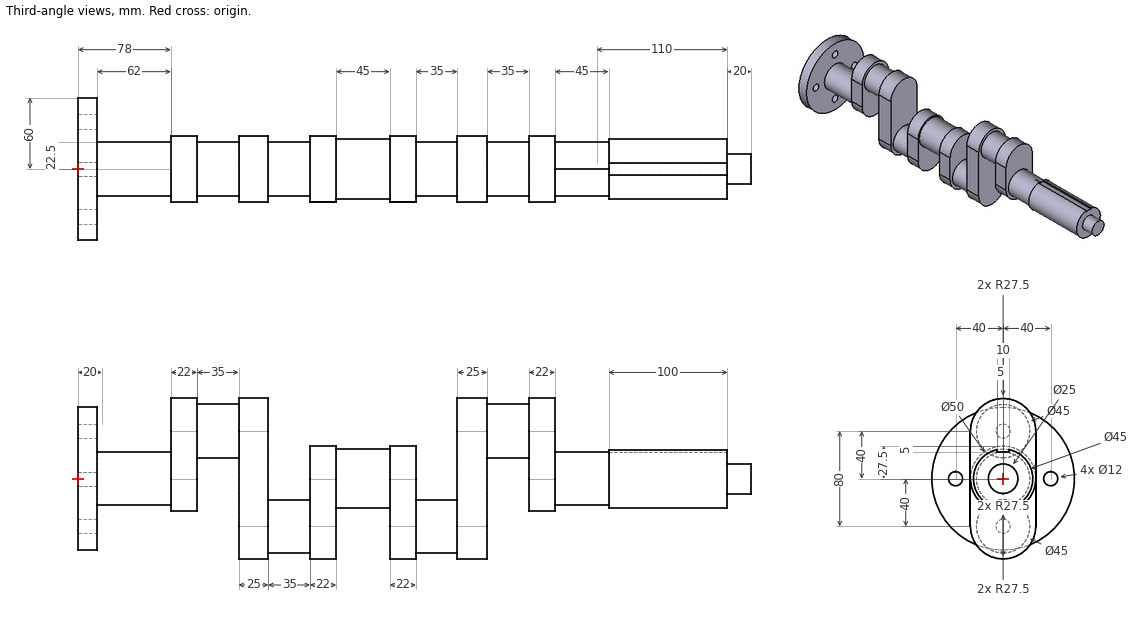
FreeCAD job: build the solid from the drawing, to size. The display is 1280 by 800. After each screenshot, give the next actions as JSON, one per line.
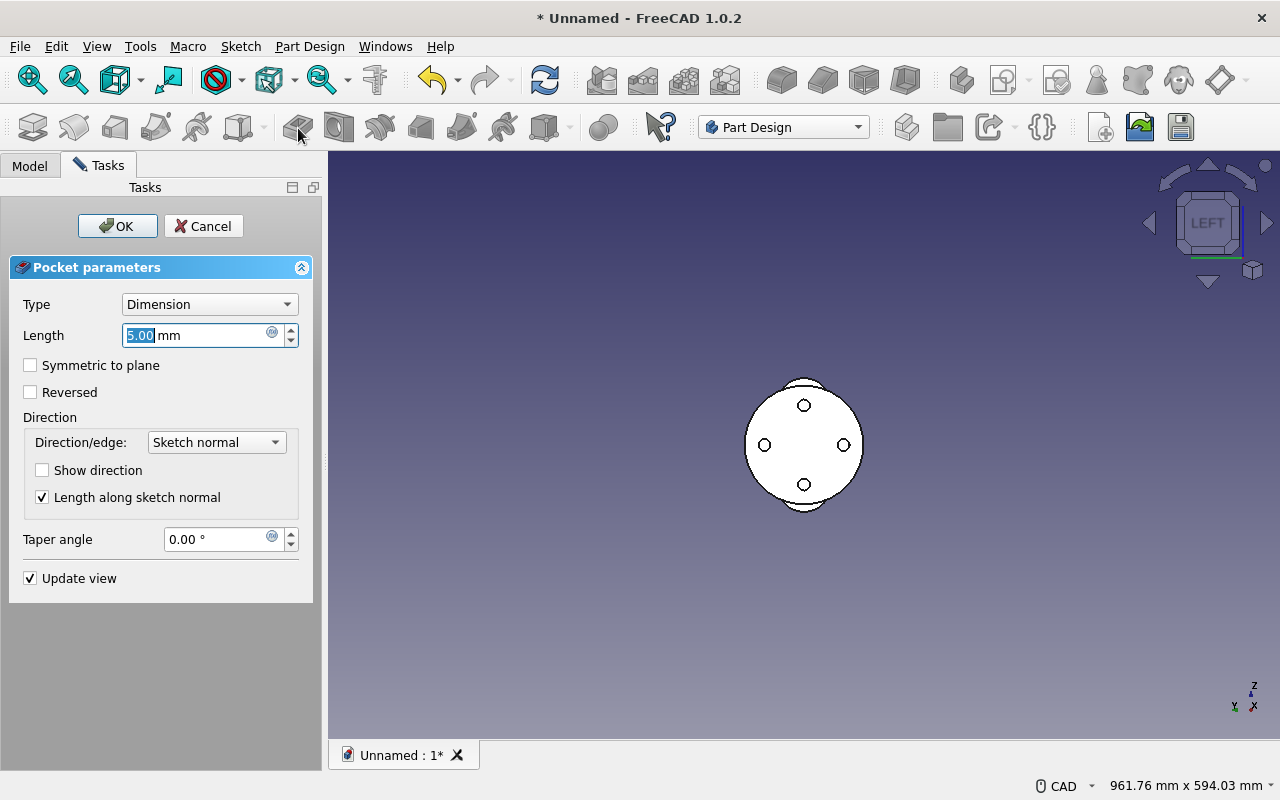
{"action": "type", "text": "20"}
{"action": "key", "text": "Tab"}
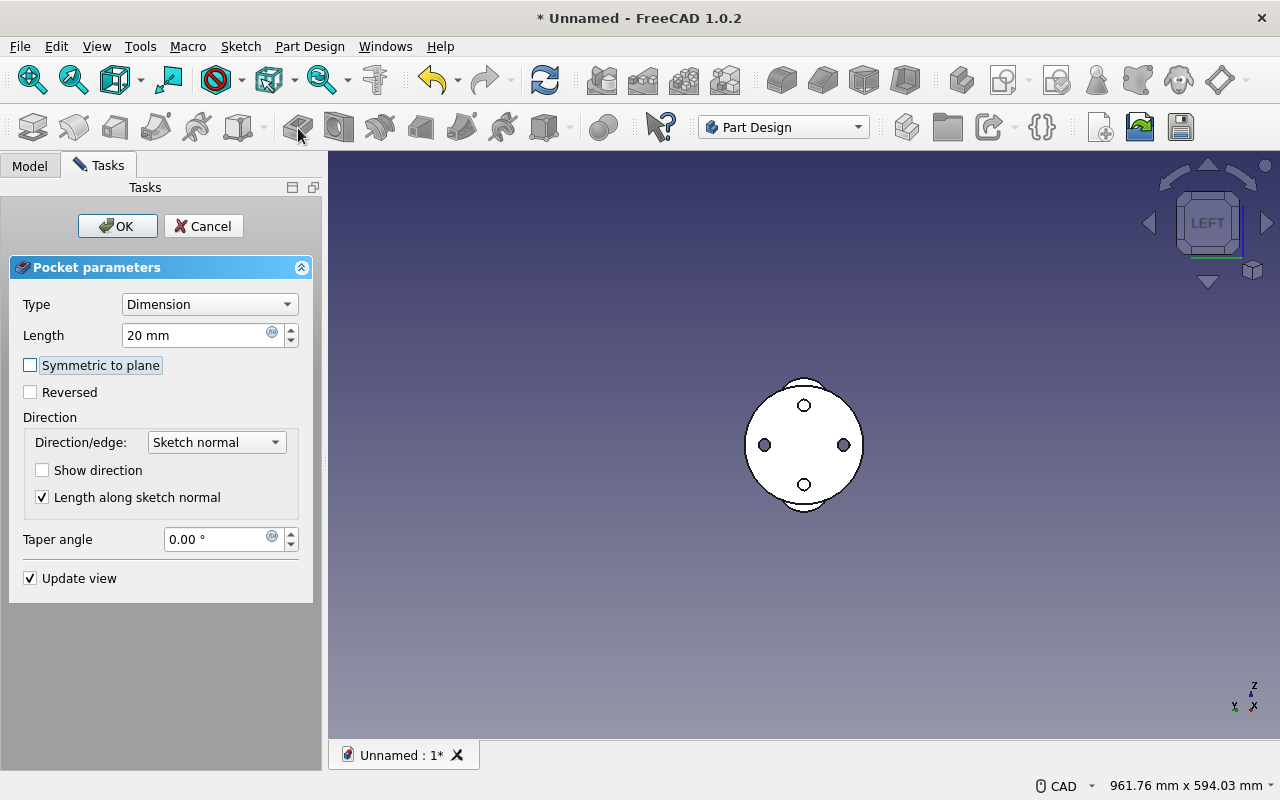
{"action": "left_click", "coordinate": [118, 226]}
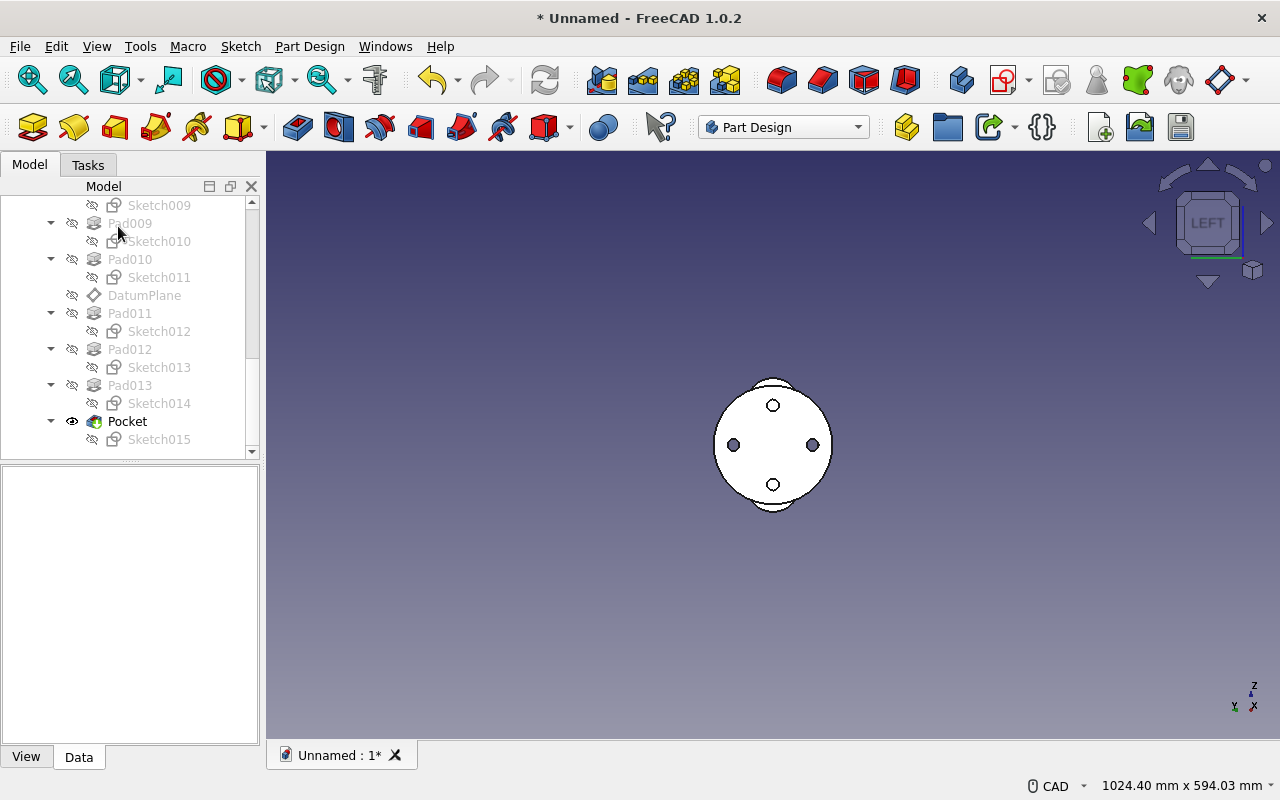
{"action": "left_click", "coordinate": [33, 80]}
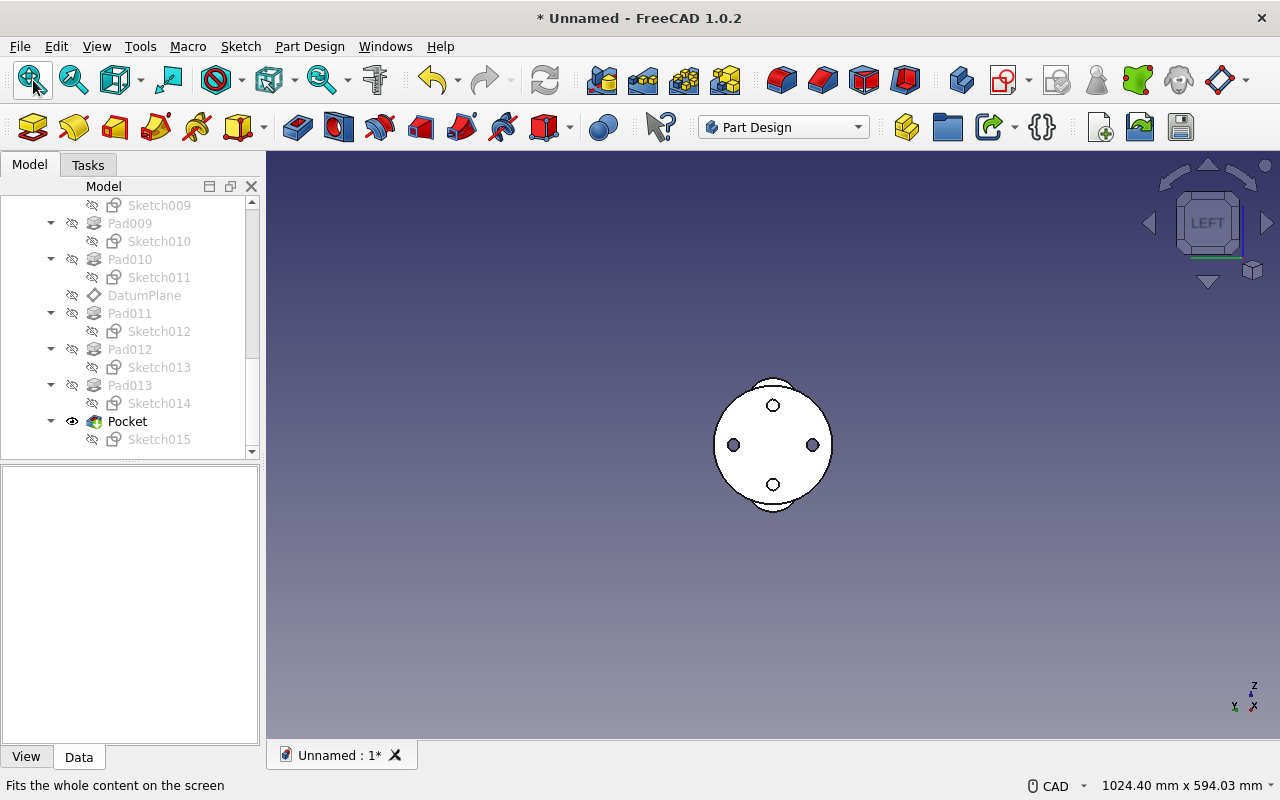
{"action": "key", "text": "0"}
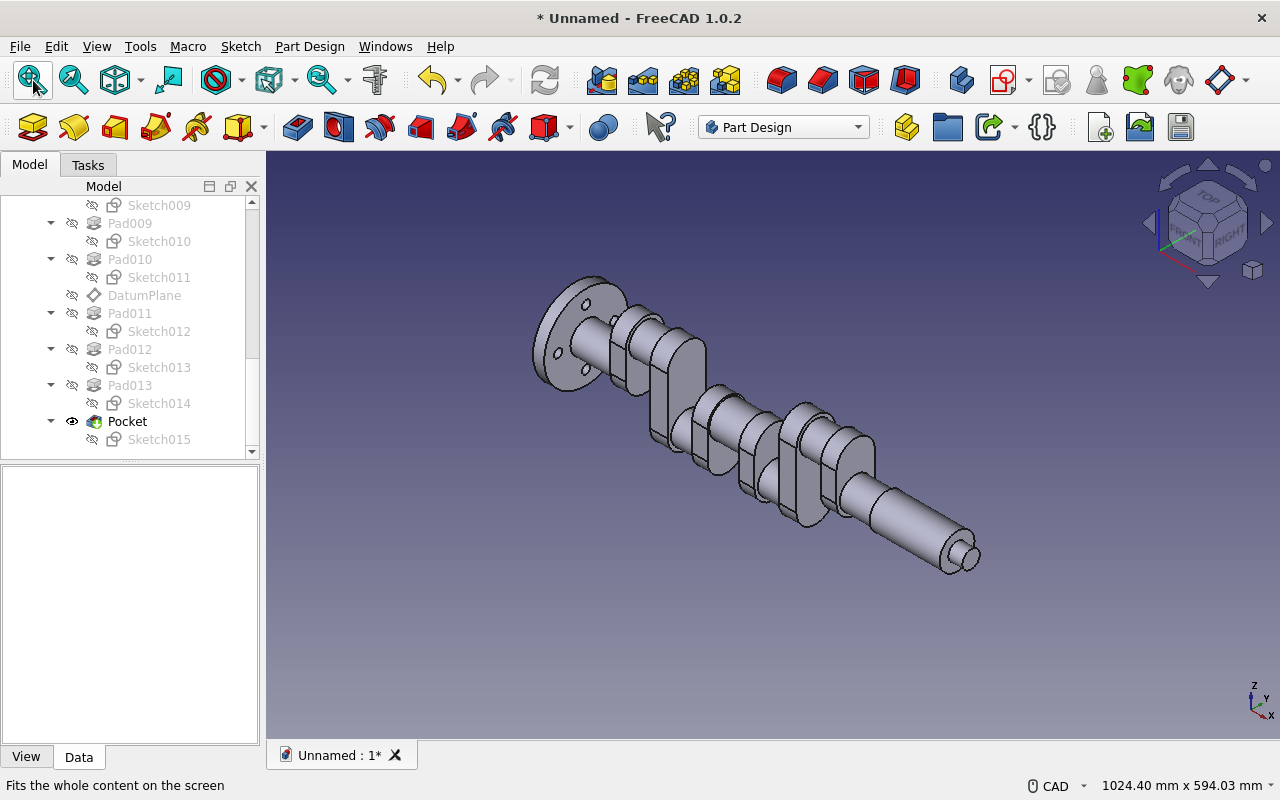
{"action": "scroll", "coordinate": [947, 568], "scroll_direction": "up", "scroll_amount": 5}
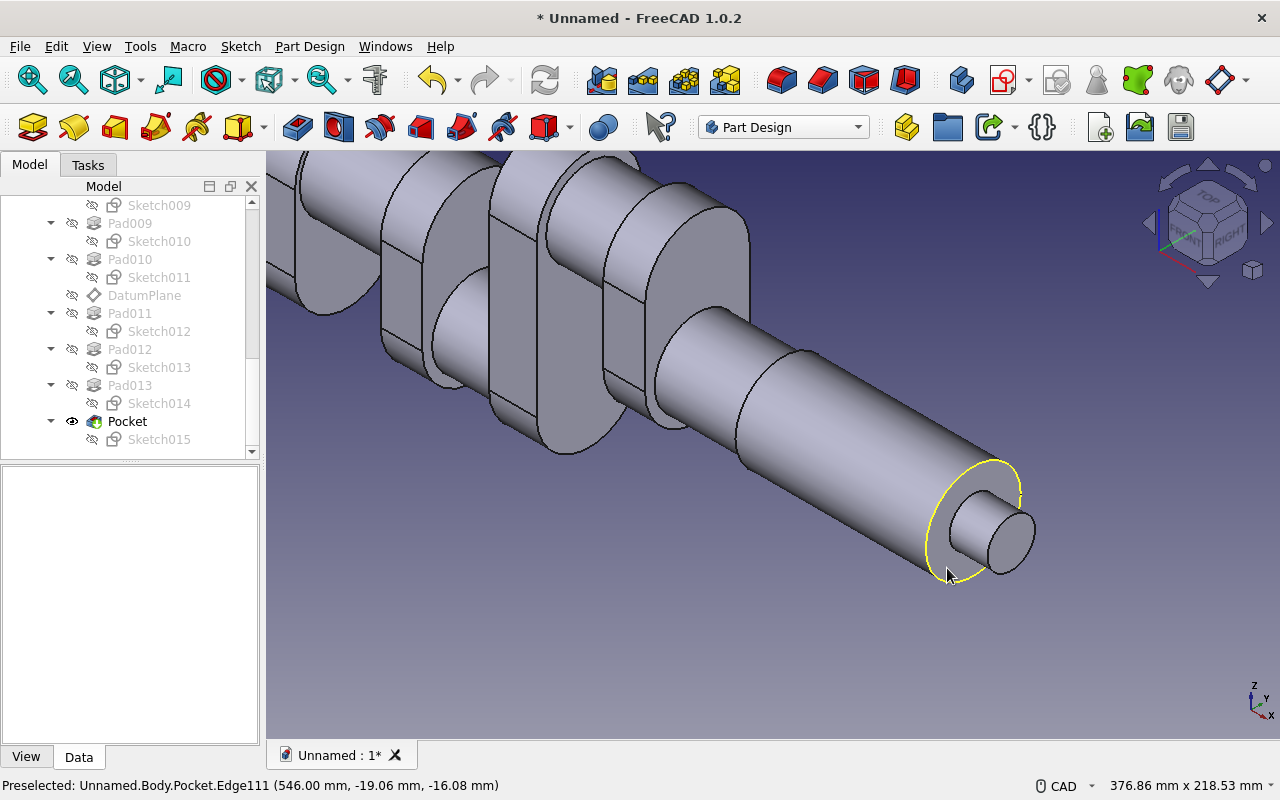
{"action": "left_click", "coordinate": [946, 567]}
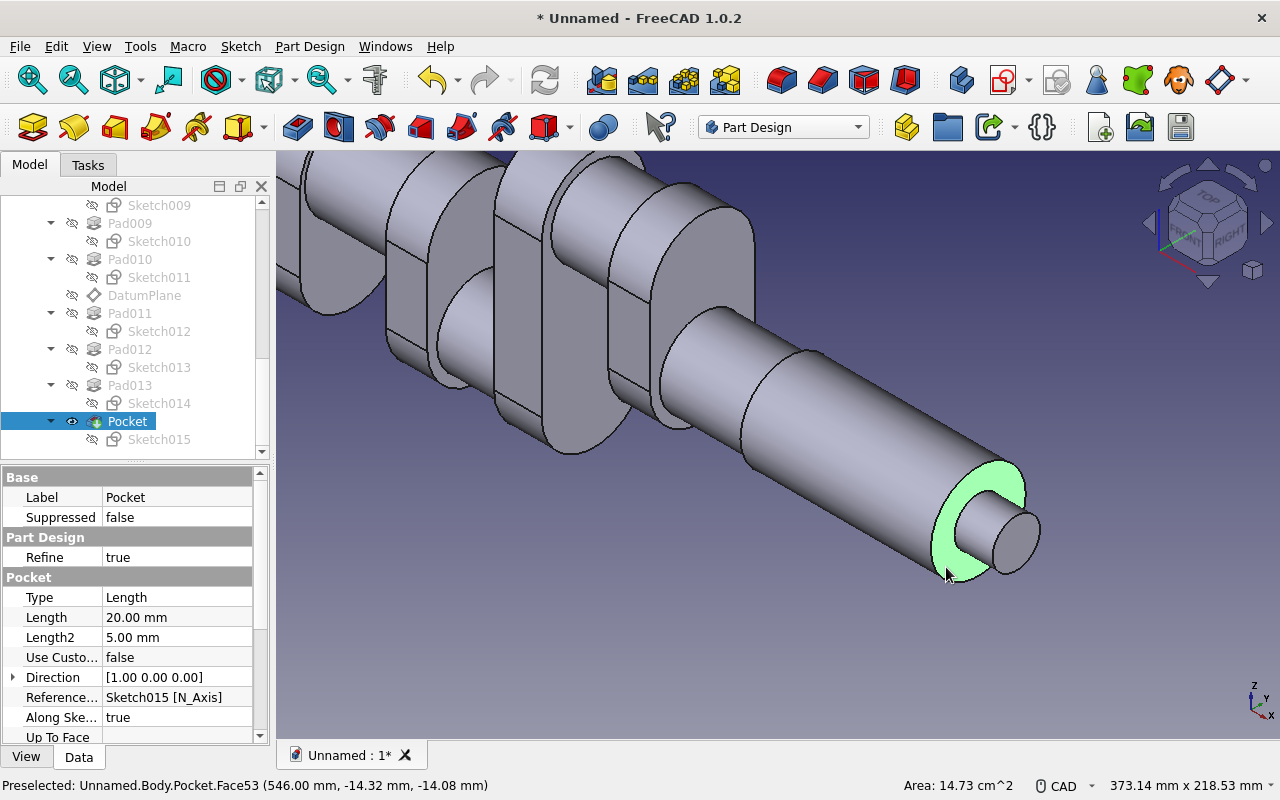
{"action": "left_click", "coordinate": [1002, 80]}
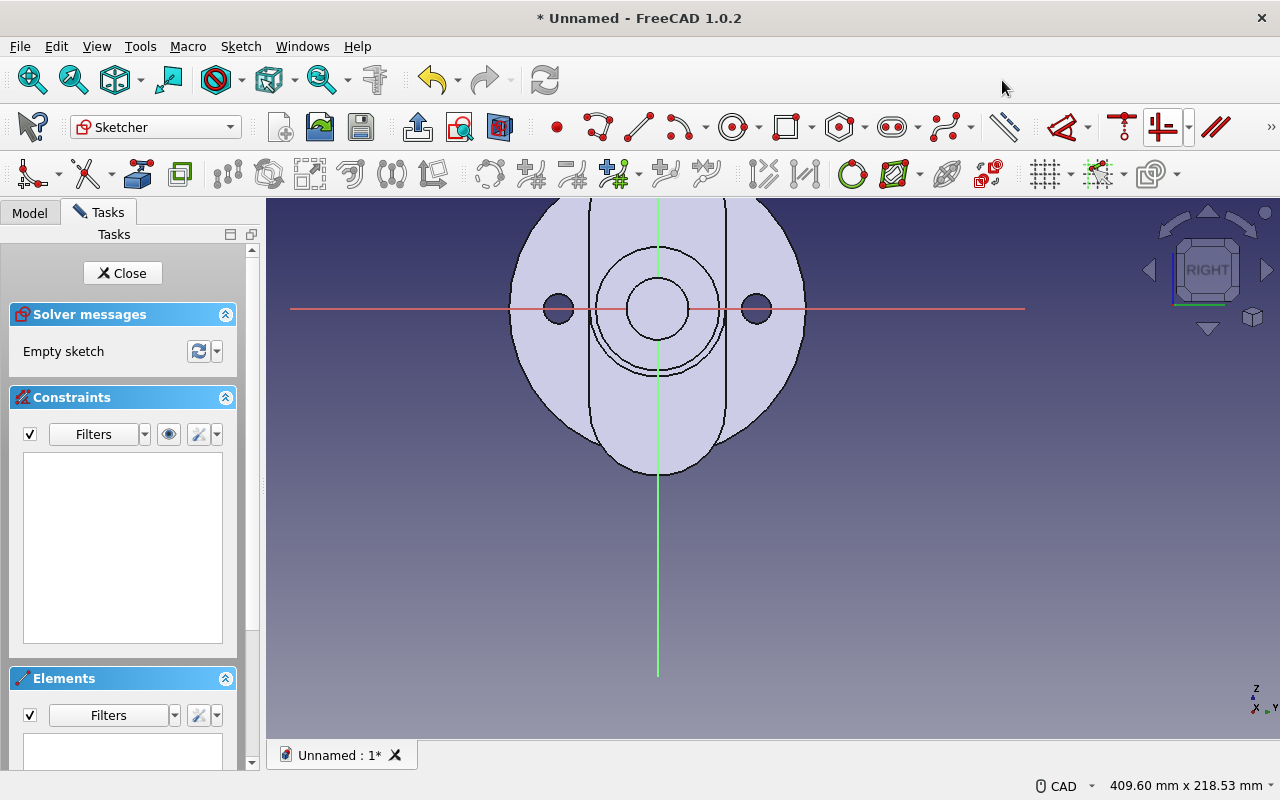
{"action": "left_click", "coordinate": [500, 128]}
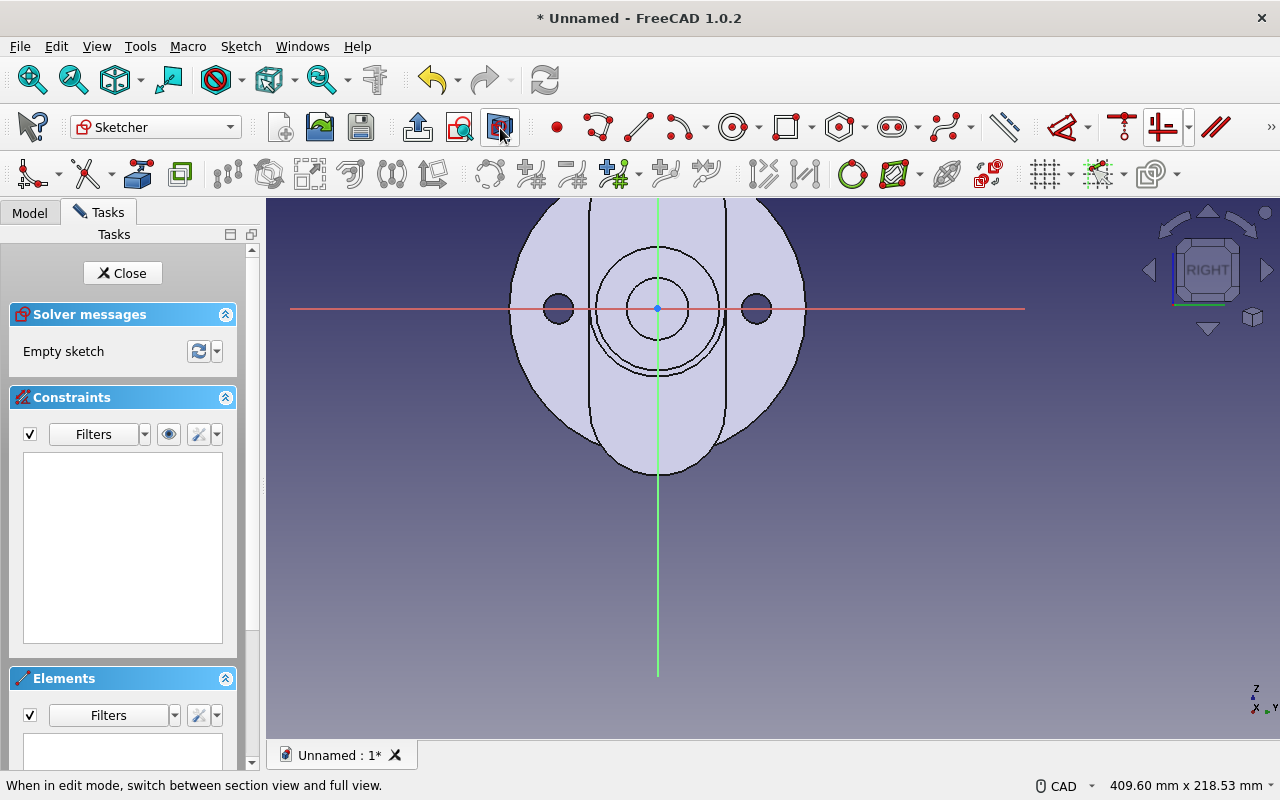
{"action": "scroll", "coordinate": [655, 235], "scroll_direction": "up", "scroll_amount": 15}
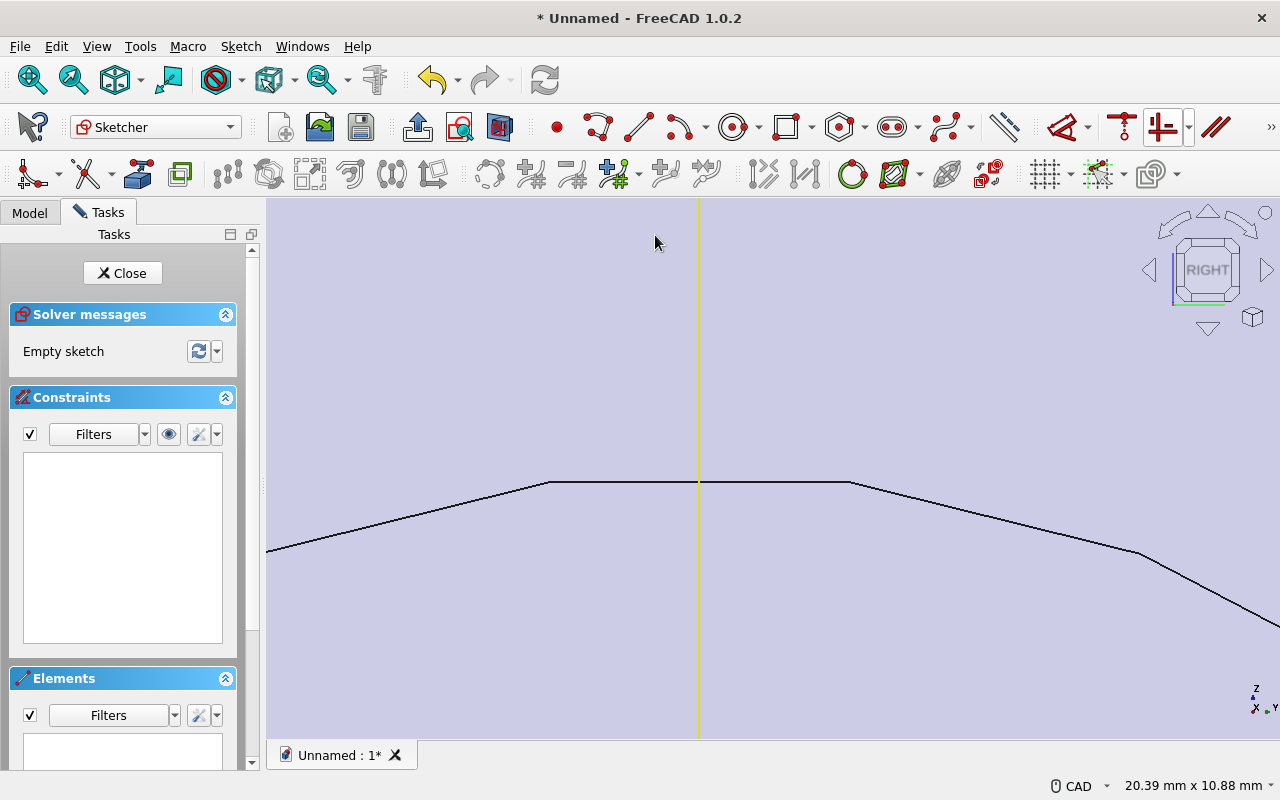
{"action": "left_click", "coordinate": [786, 128]}